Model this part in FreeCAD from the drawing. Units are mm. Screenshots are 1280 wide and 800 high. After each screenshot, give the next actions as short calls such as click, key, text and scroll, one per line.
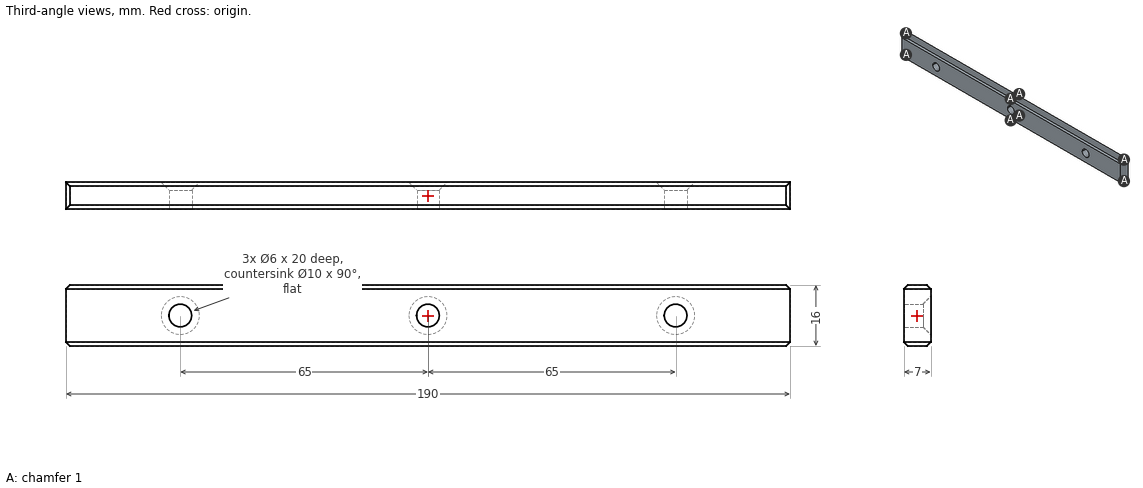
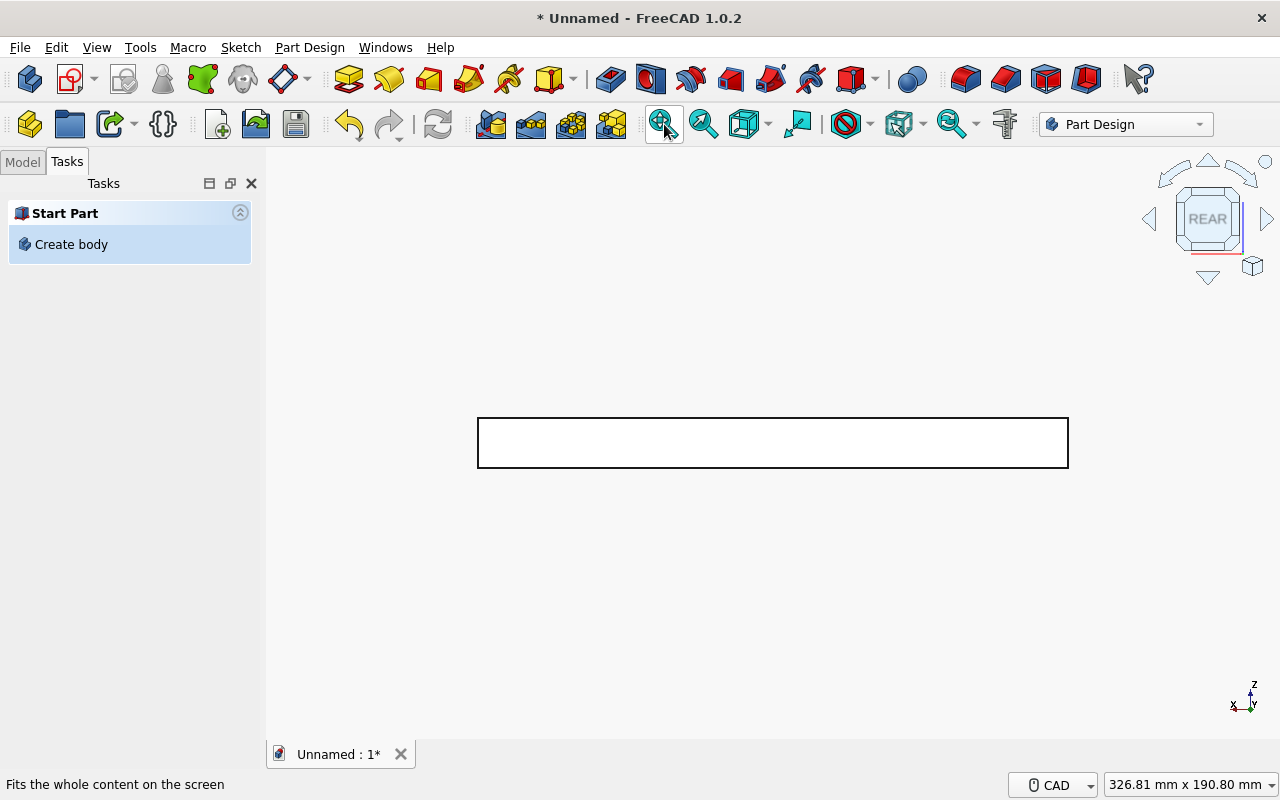
click(520, 442)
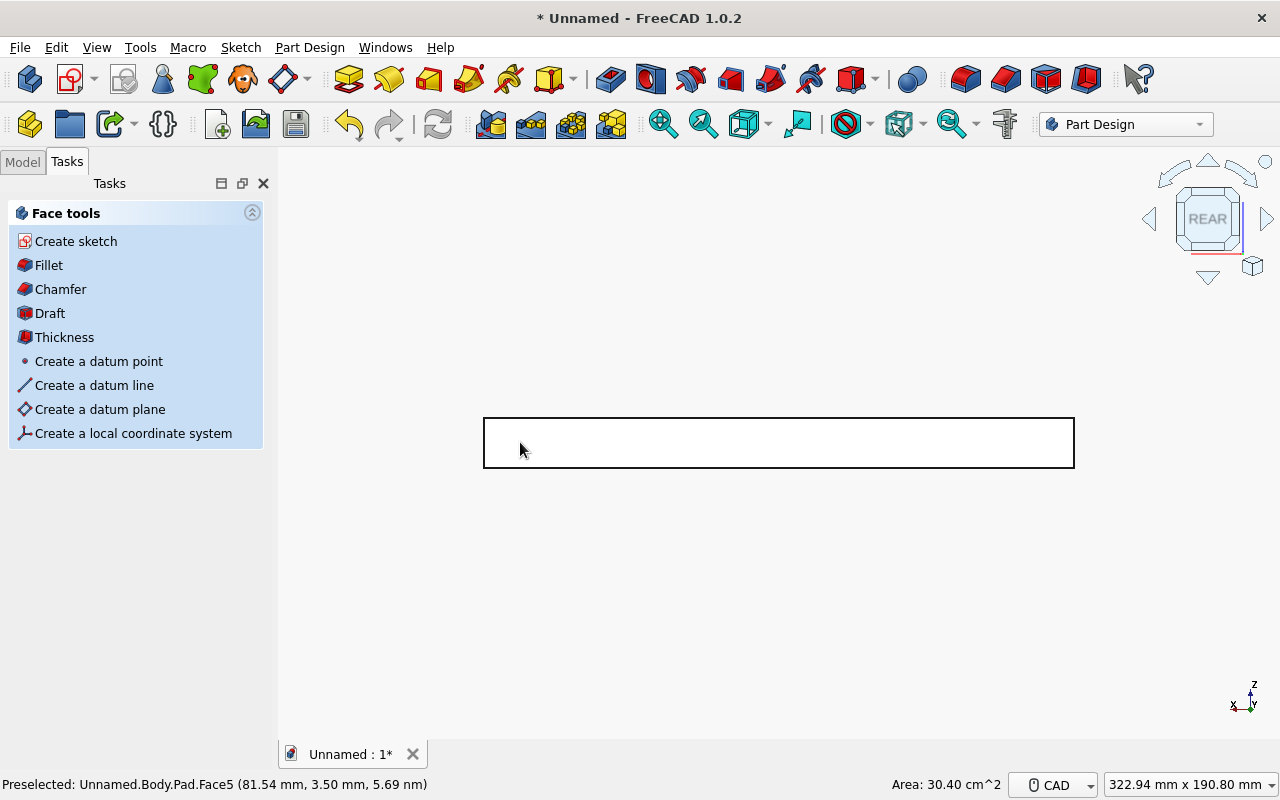
click(70, 80)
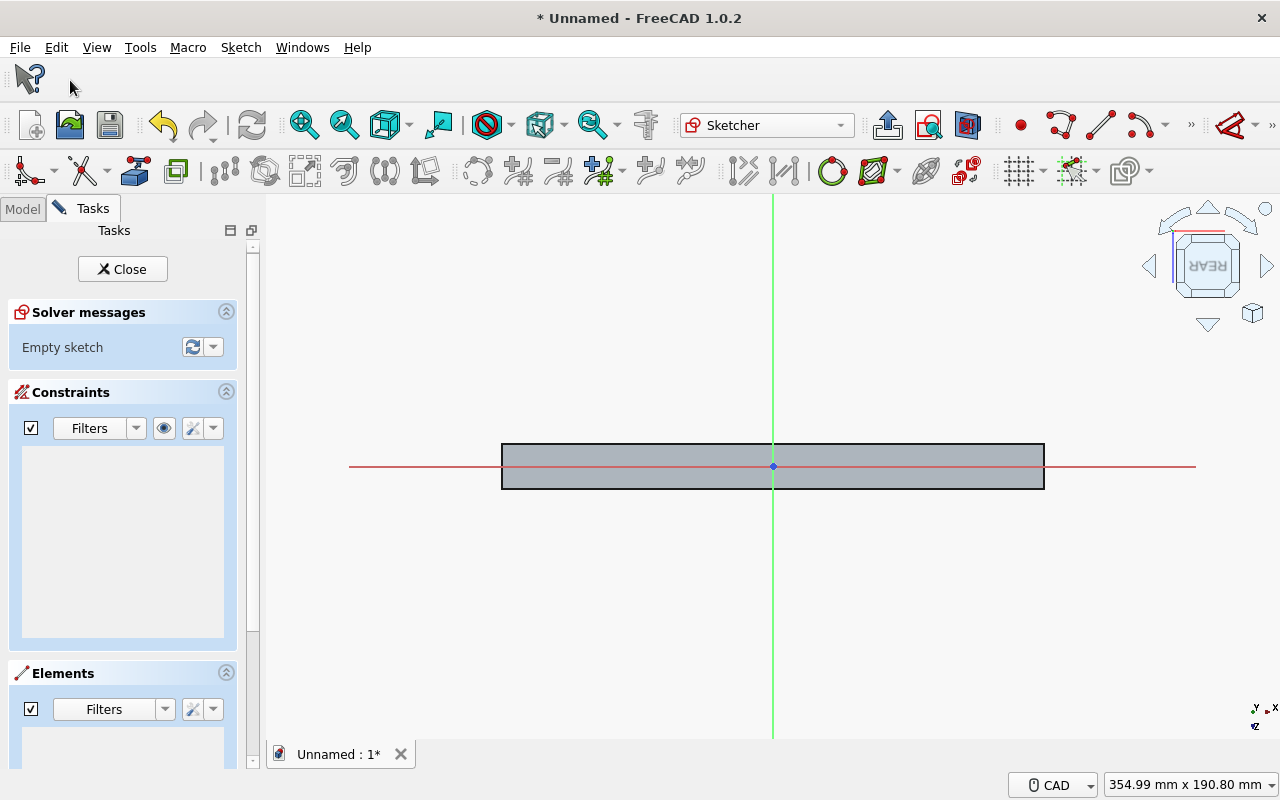
scroll(912, 466, up, 2)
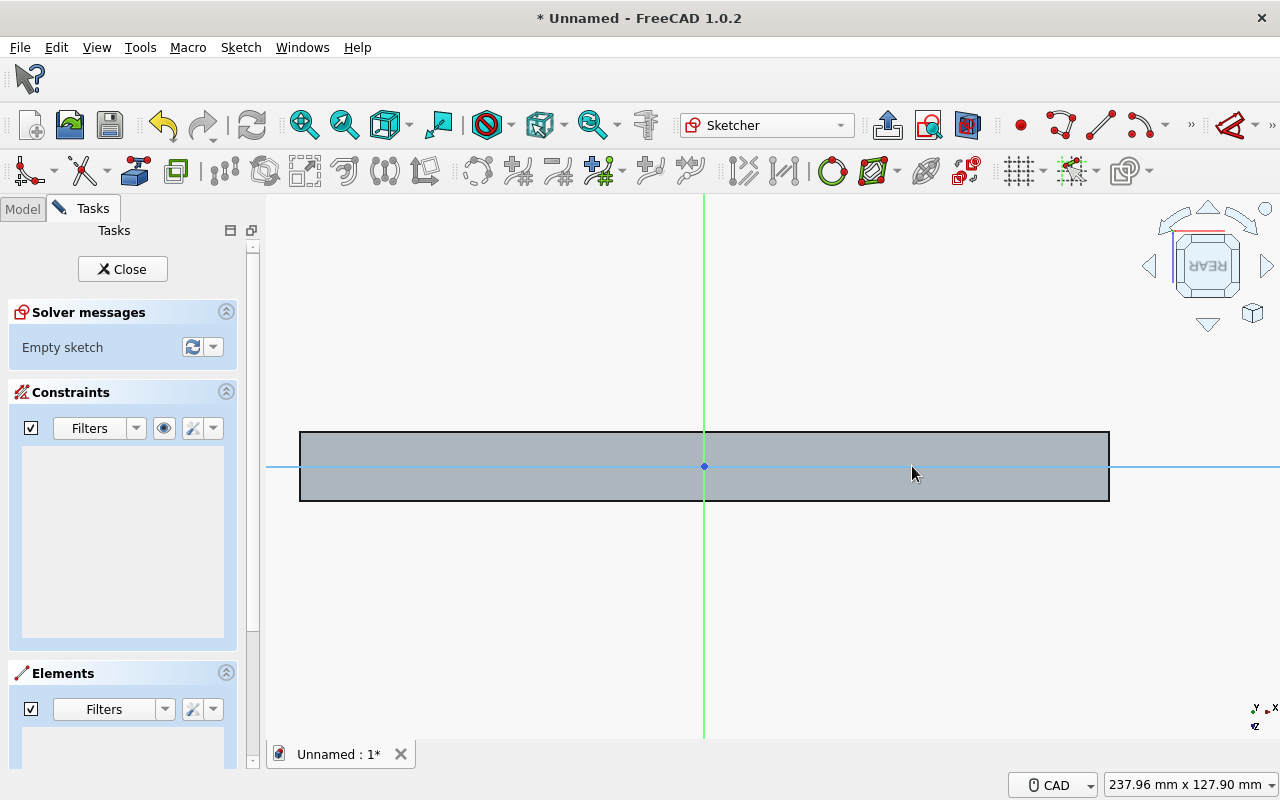
key(g)
key(c)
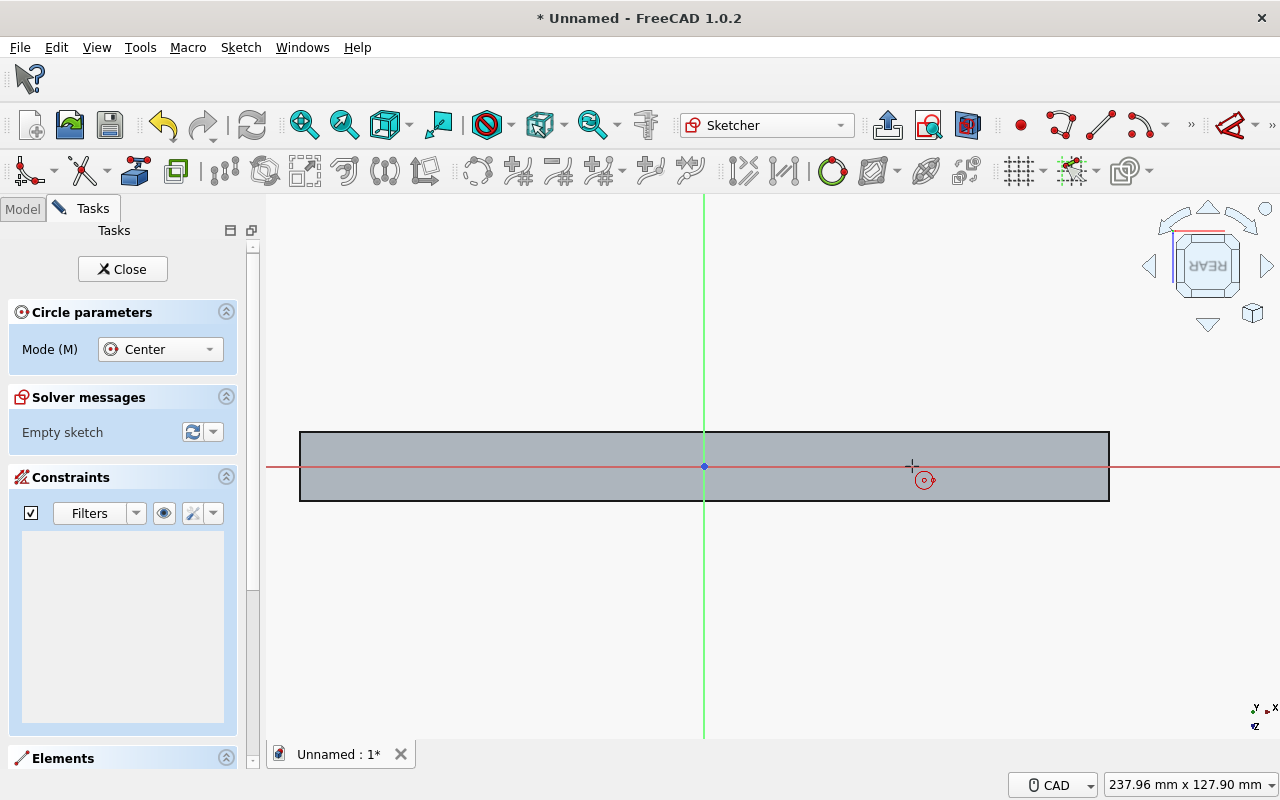
scroll(427, 466, up, 3)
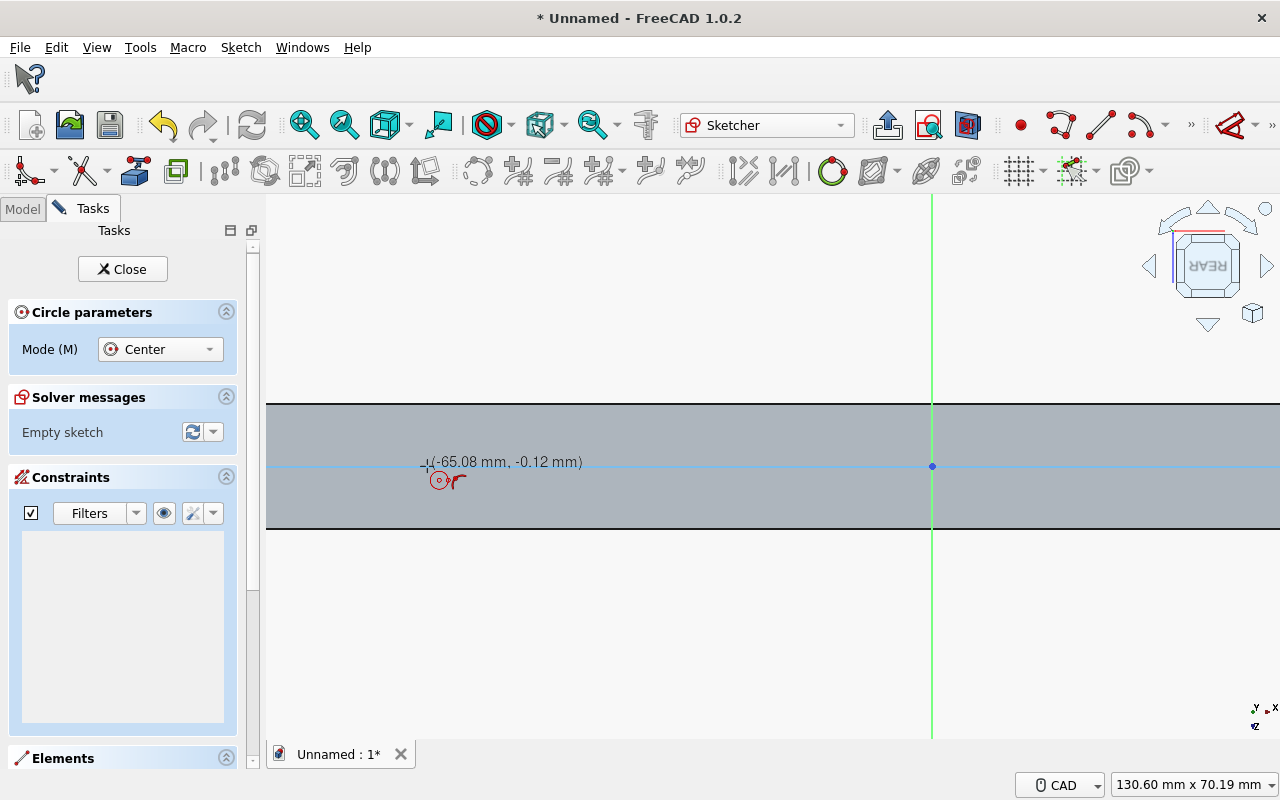
click(427, 466)
click(444, 450)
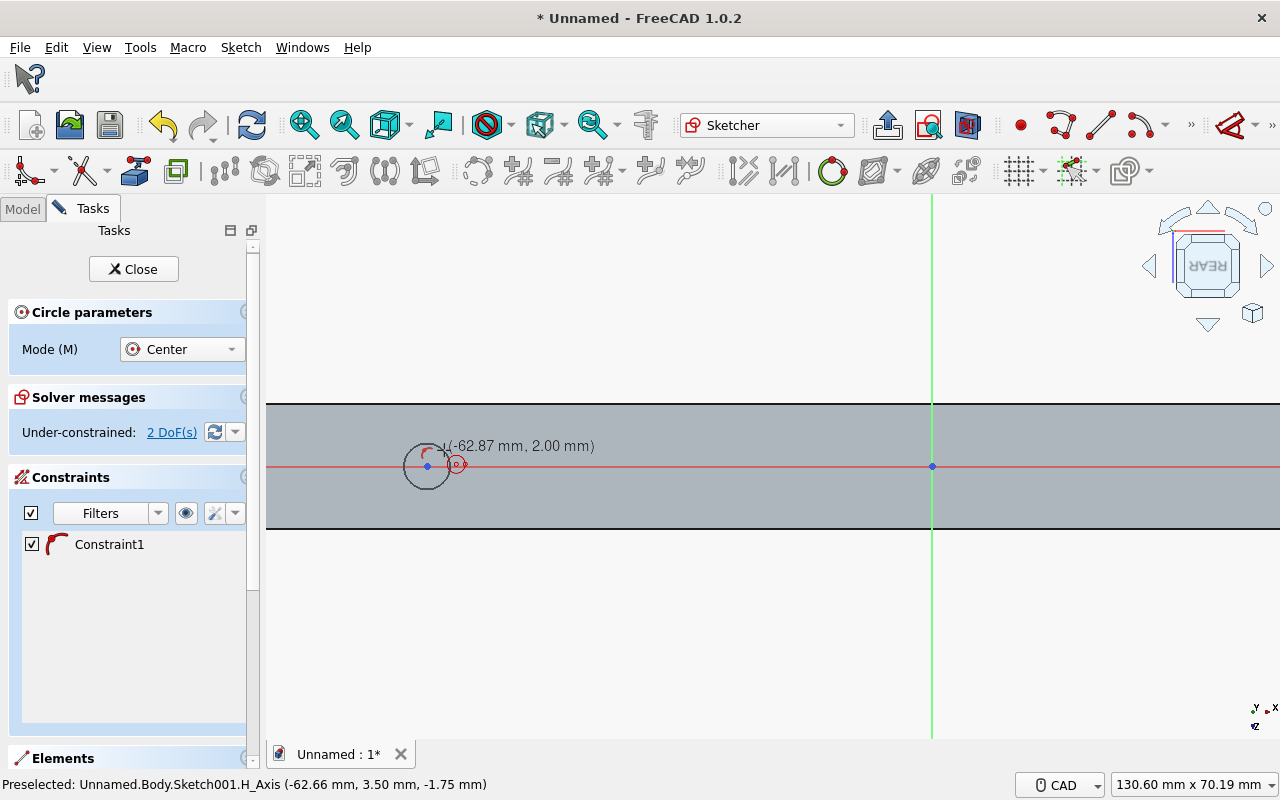
click(932, 466)
click(949, 450)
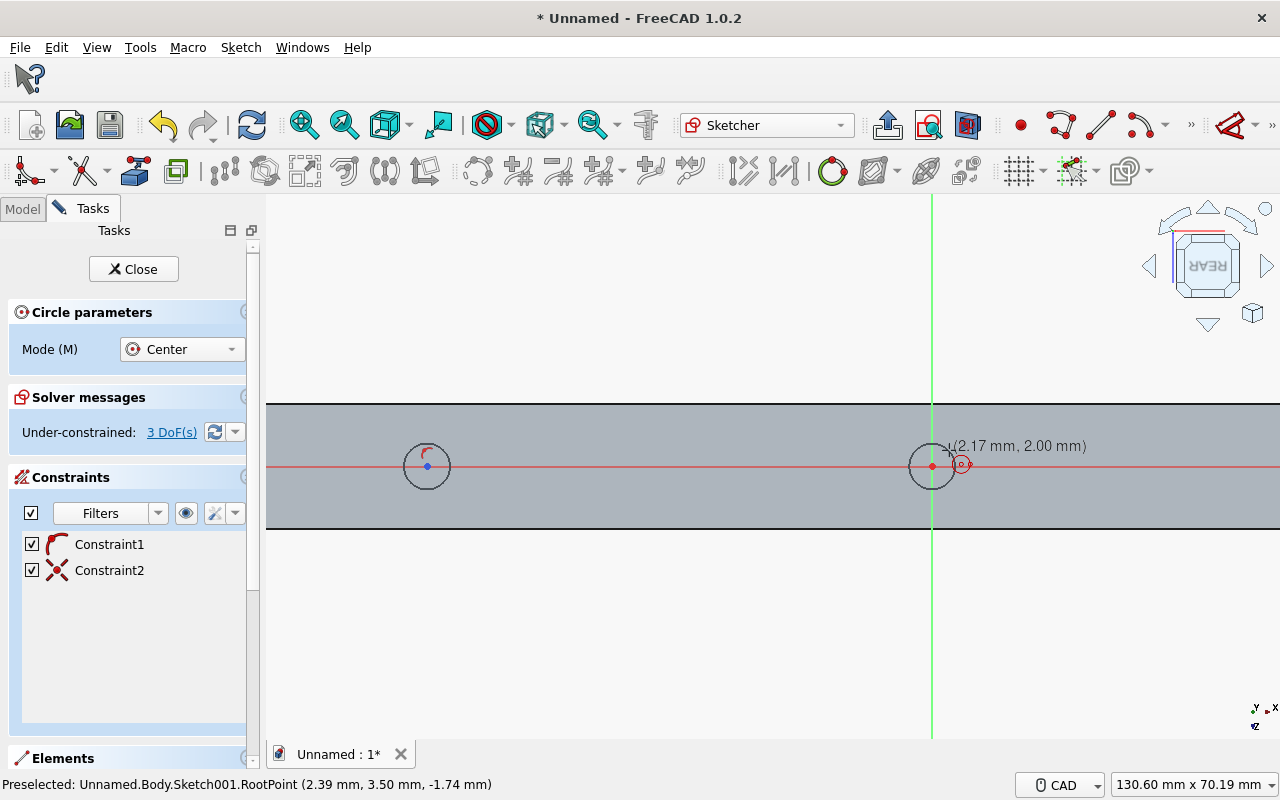
scroll(428, 467, down, 3)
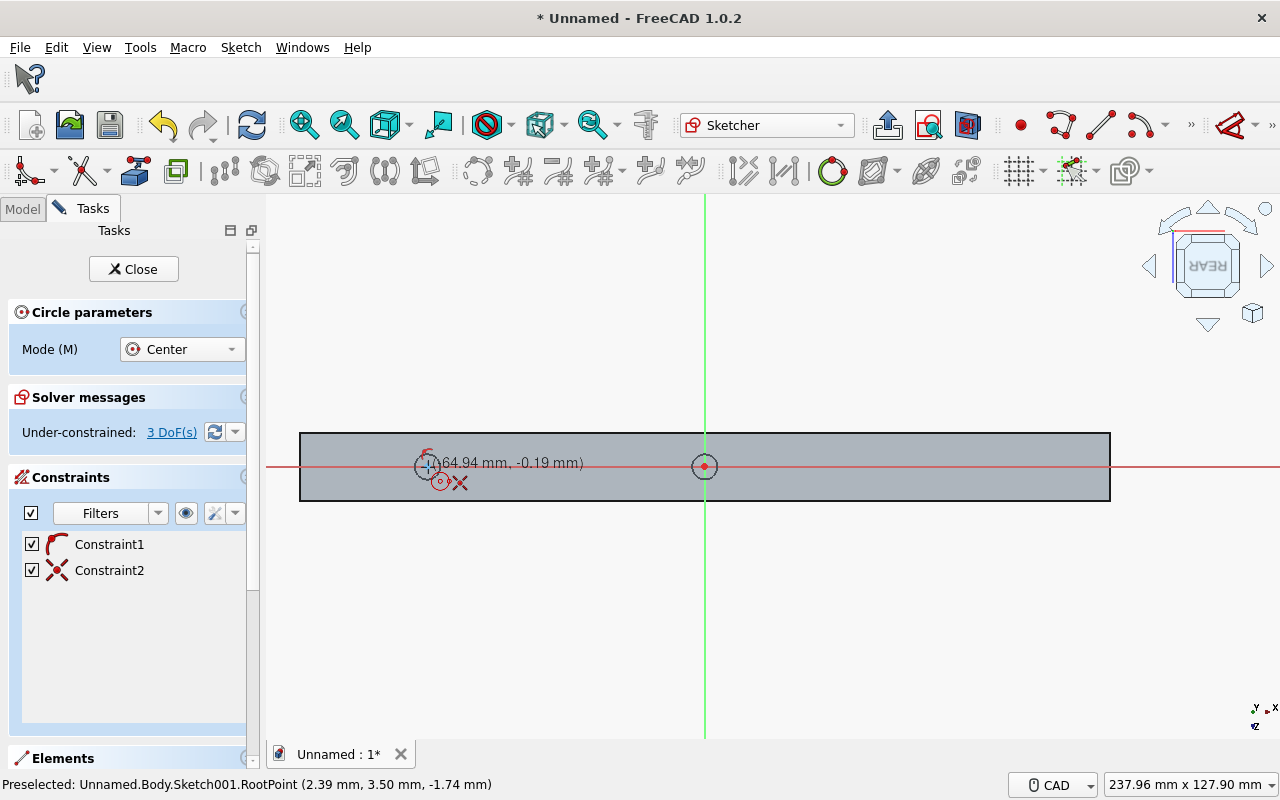
scroll(982, 467, up, 3)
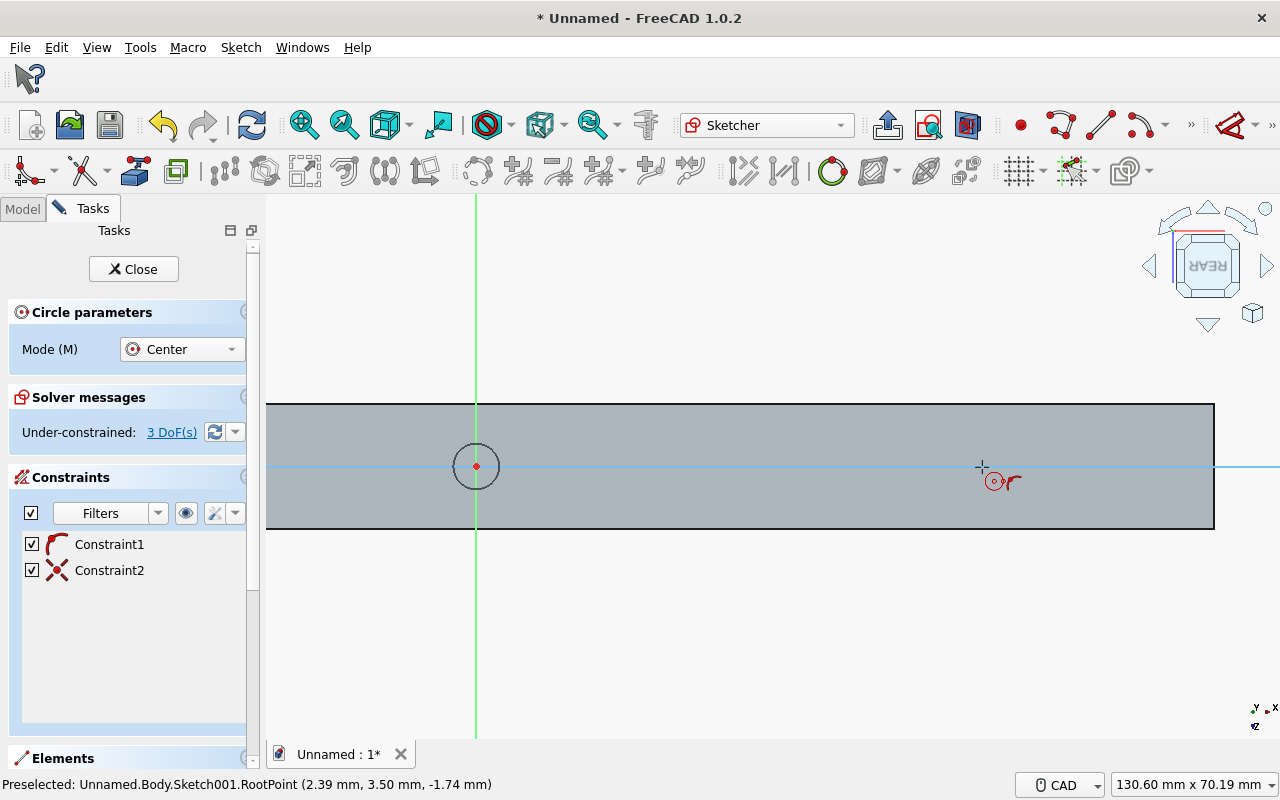
click(981, 466)
click(997, 450)
key(Escape)